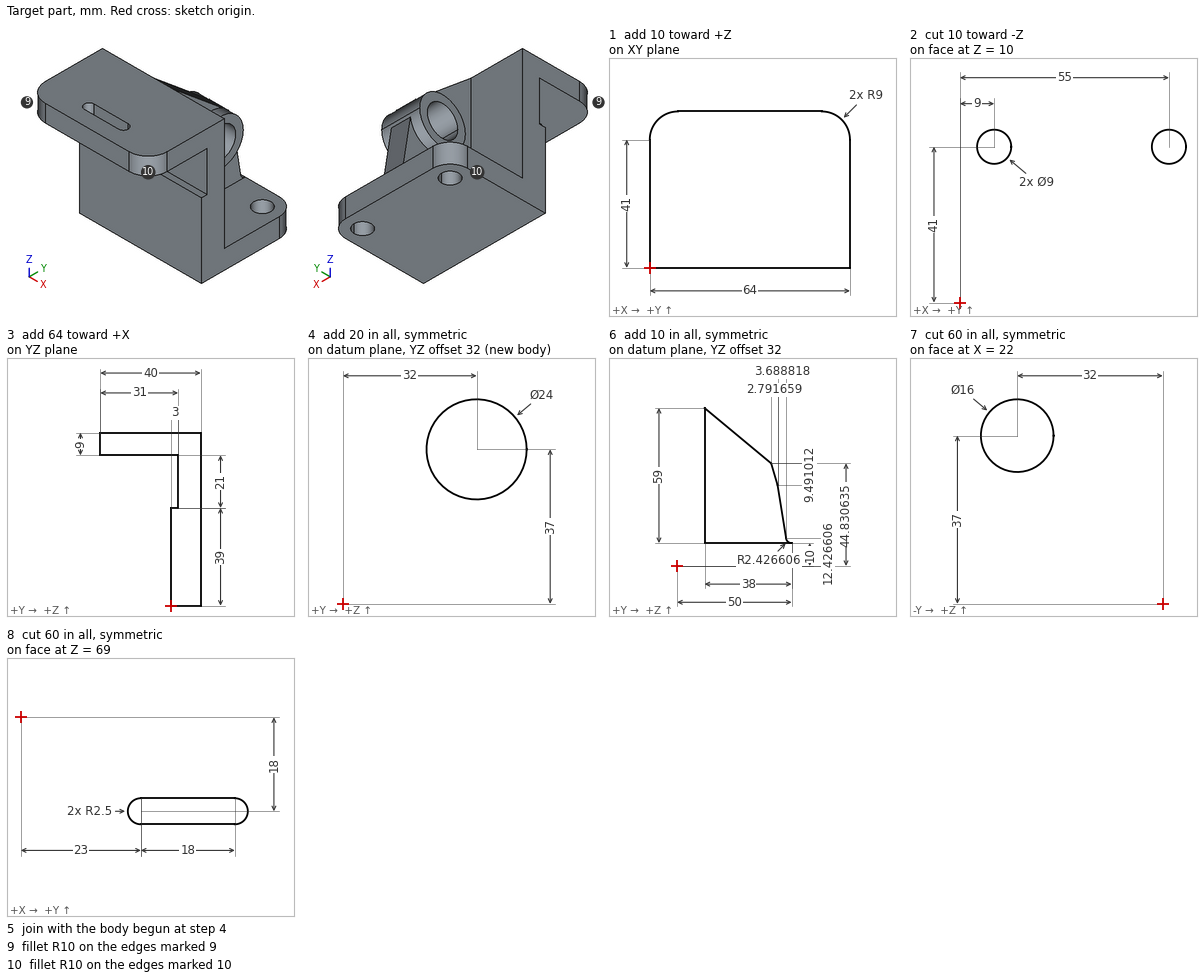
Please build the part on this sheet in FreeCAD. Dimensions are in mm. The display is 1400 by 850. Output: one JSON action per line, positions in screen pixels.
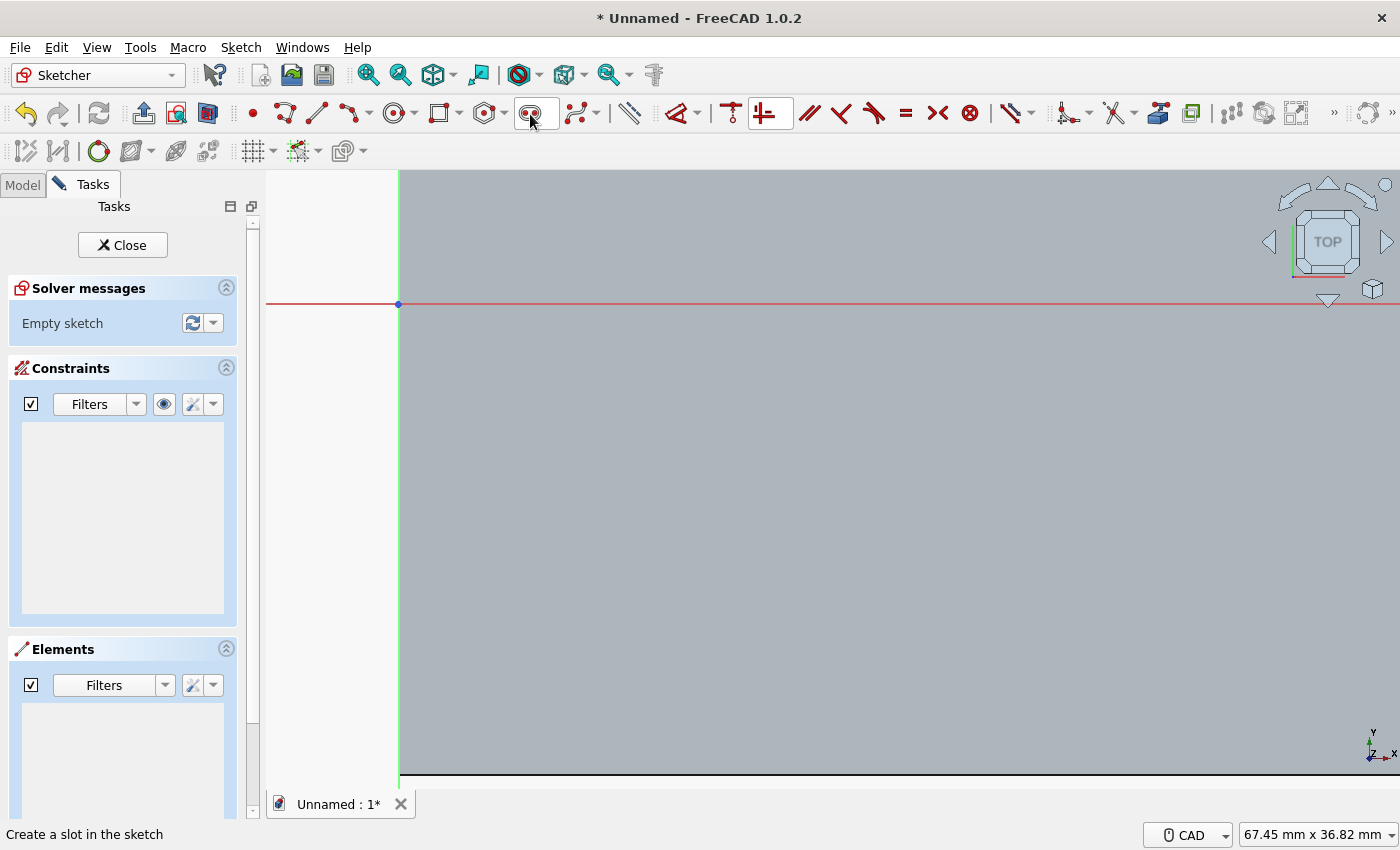
{"action": "left_click", "coordinate": [785, 607]}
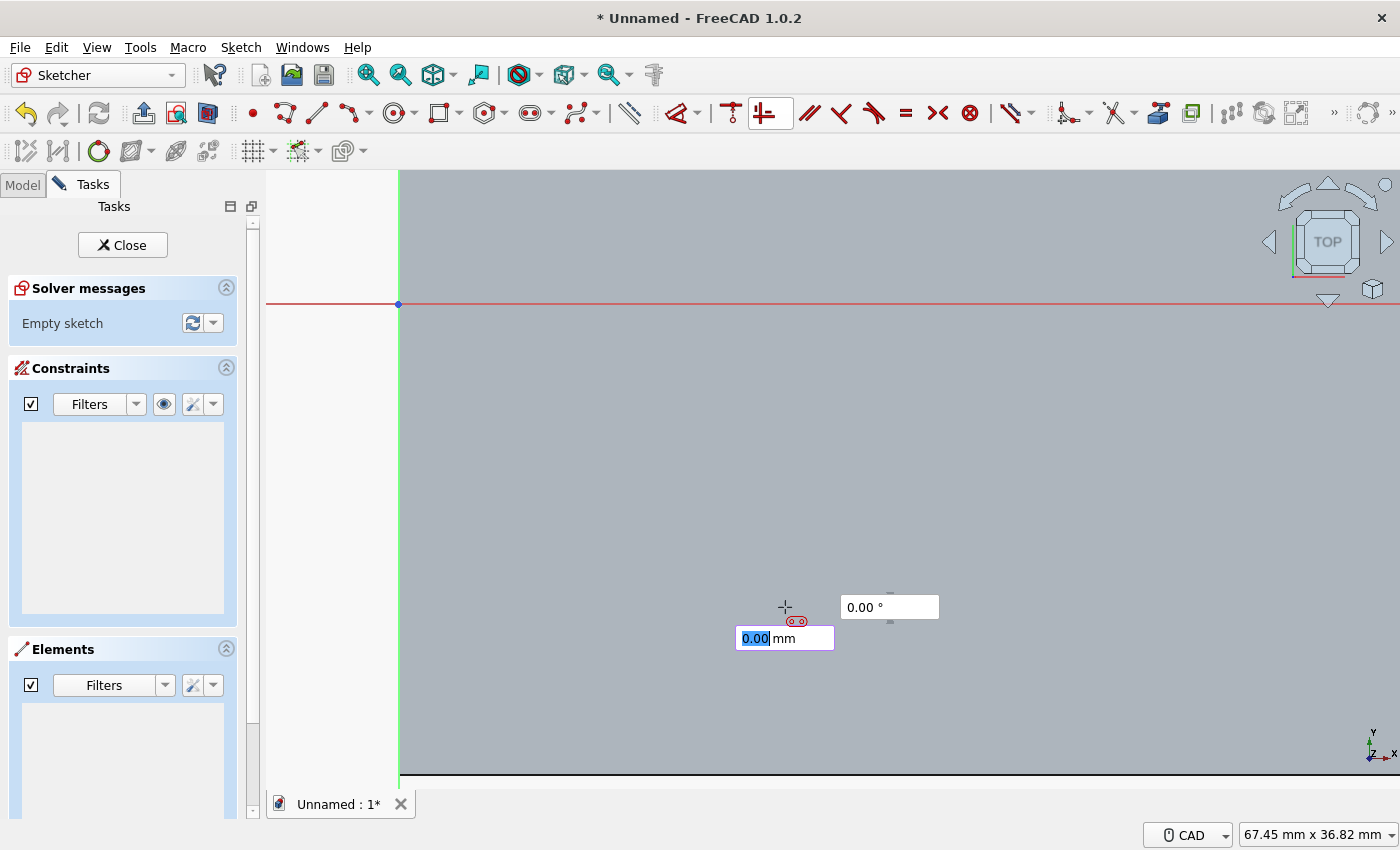
{"action": "left_click", "coordinate": [1088, 607]}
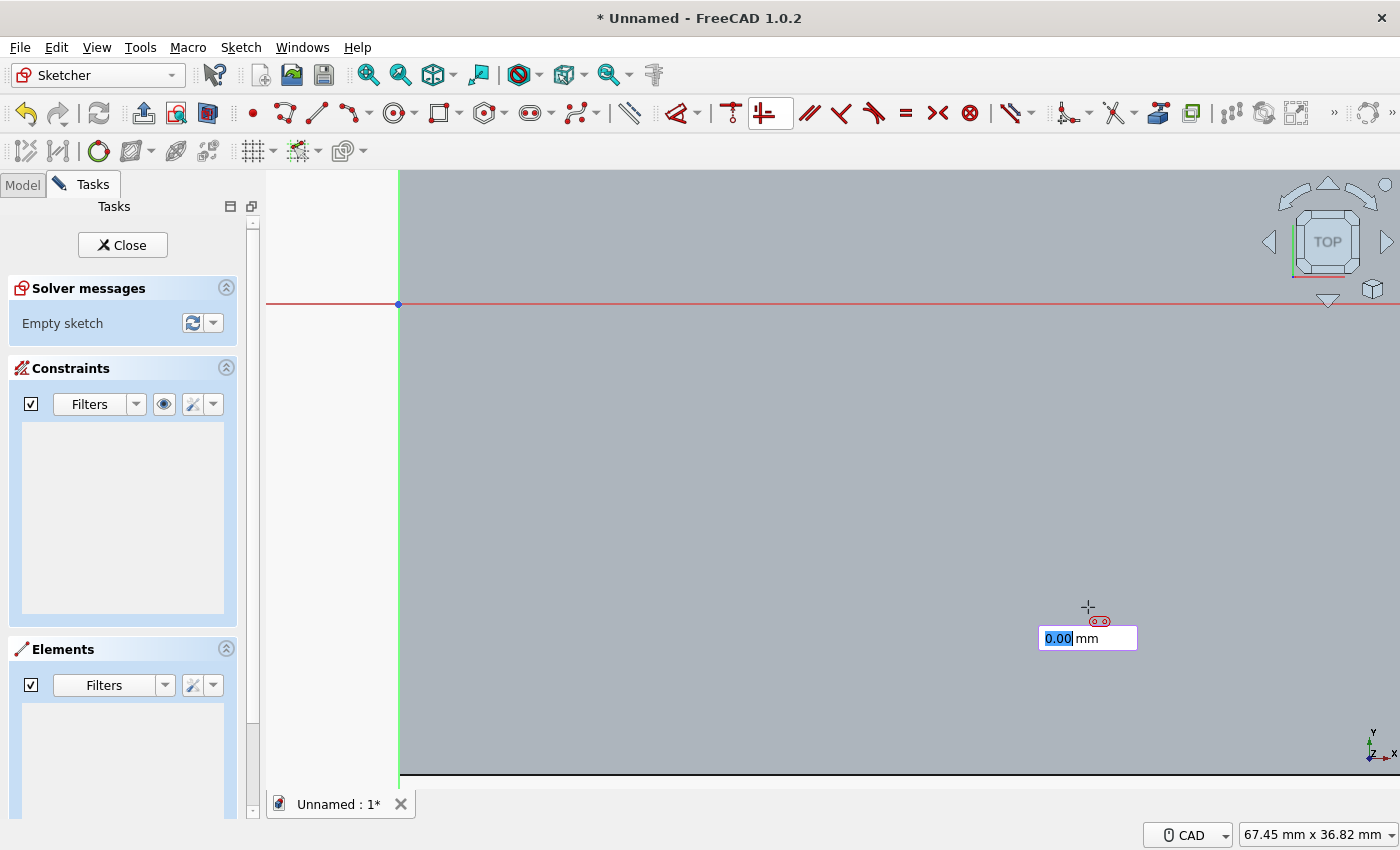
{"action": "left_click", "coordinate": [937, 565]}
{"action": "key", "text": "Escape"}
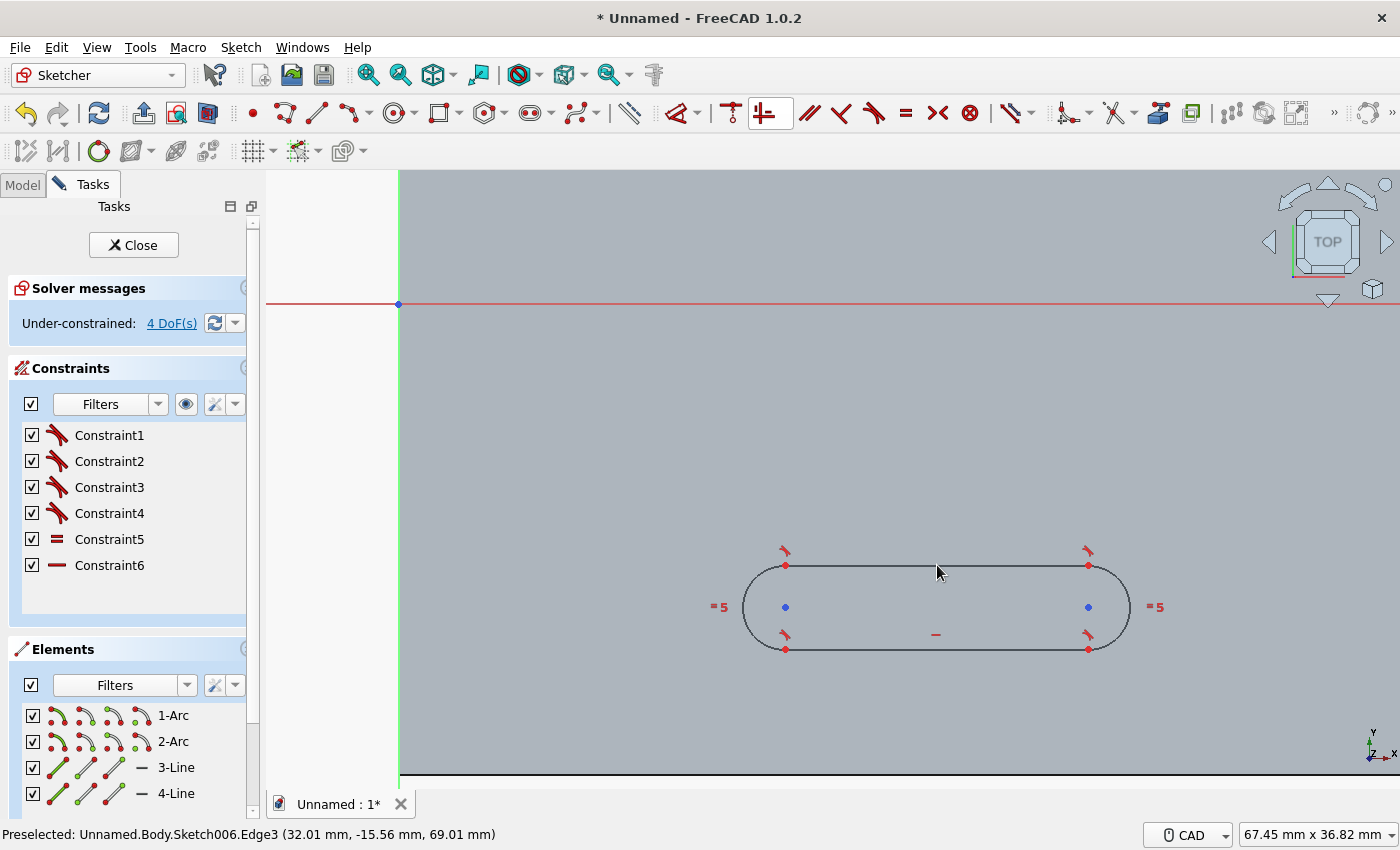
{"action": "left_click", "coordinate": [676, 114]}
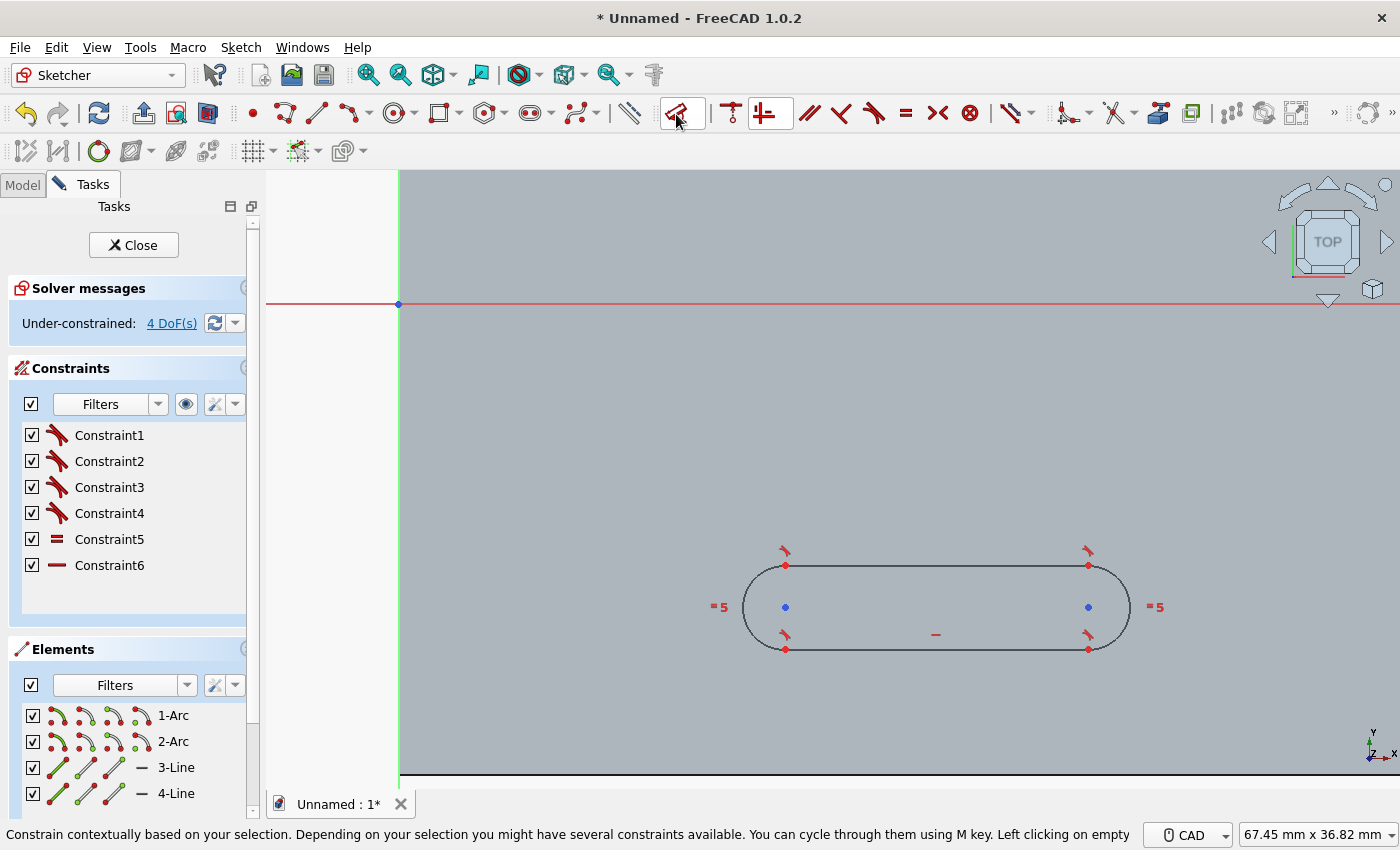
{"action": "left_click", "coordinate": [751, 583]}
{"action": "left_click", "coordinate": [725, 564]}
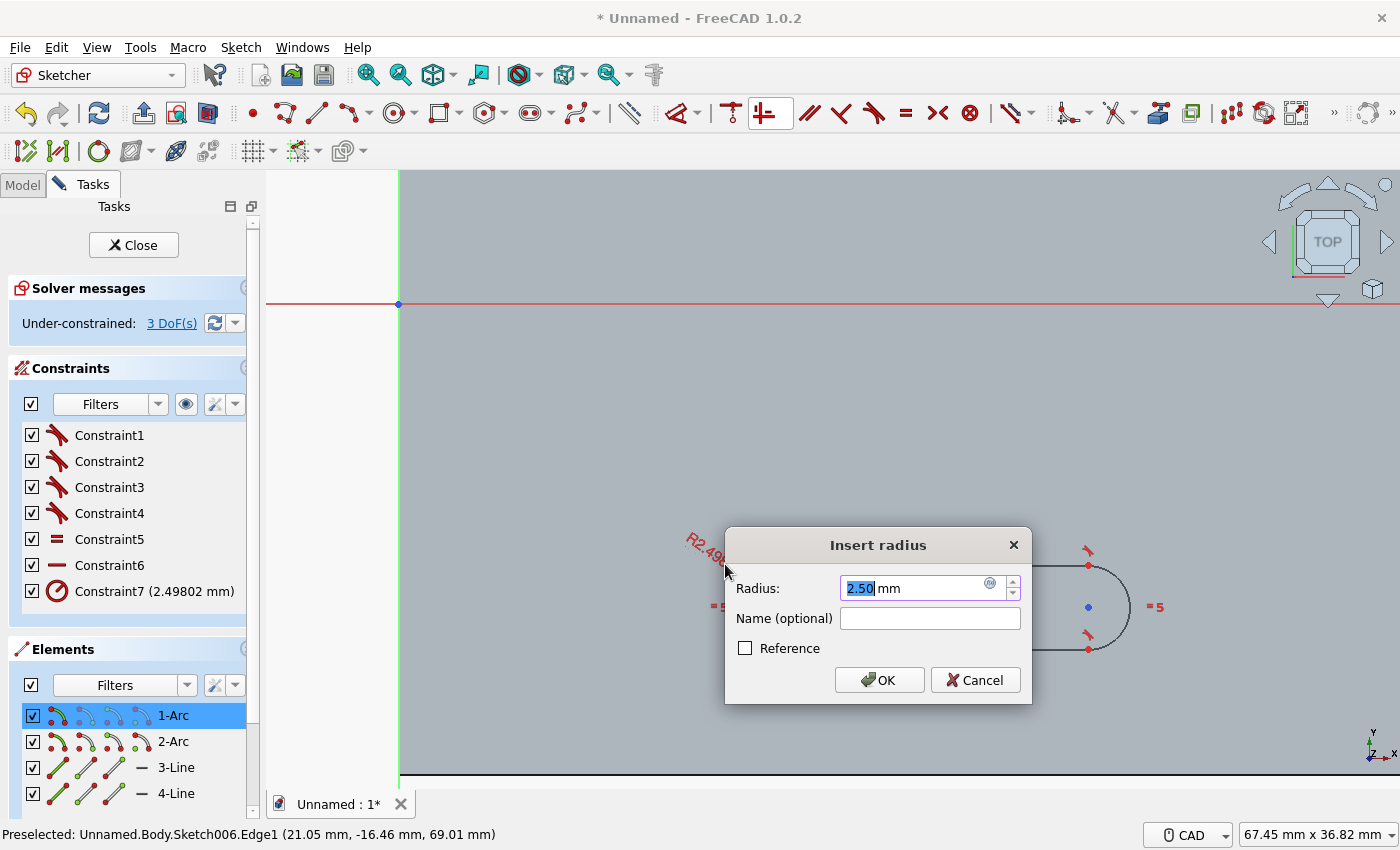
{"action": "type", "text": "2.5"}
{"action": "key", "text": "Return"}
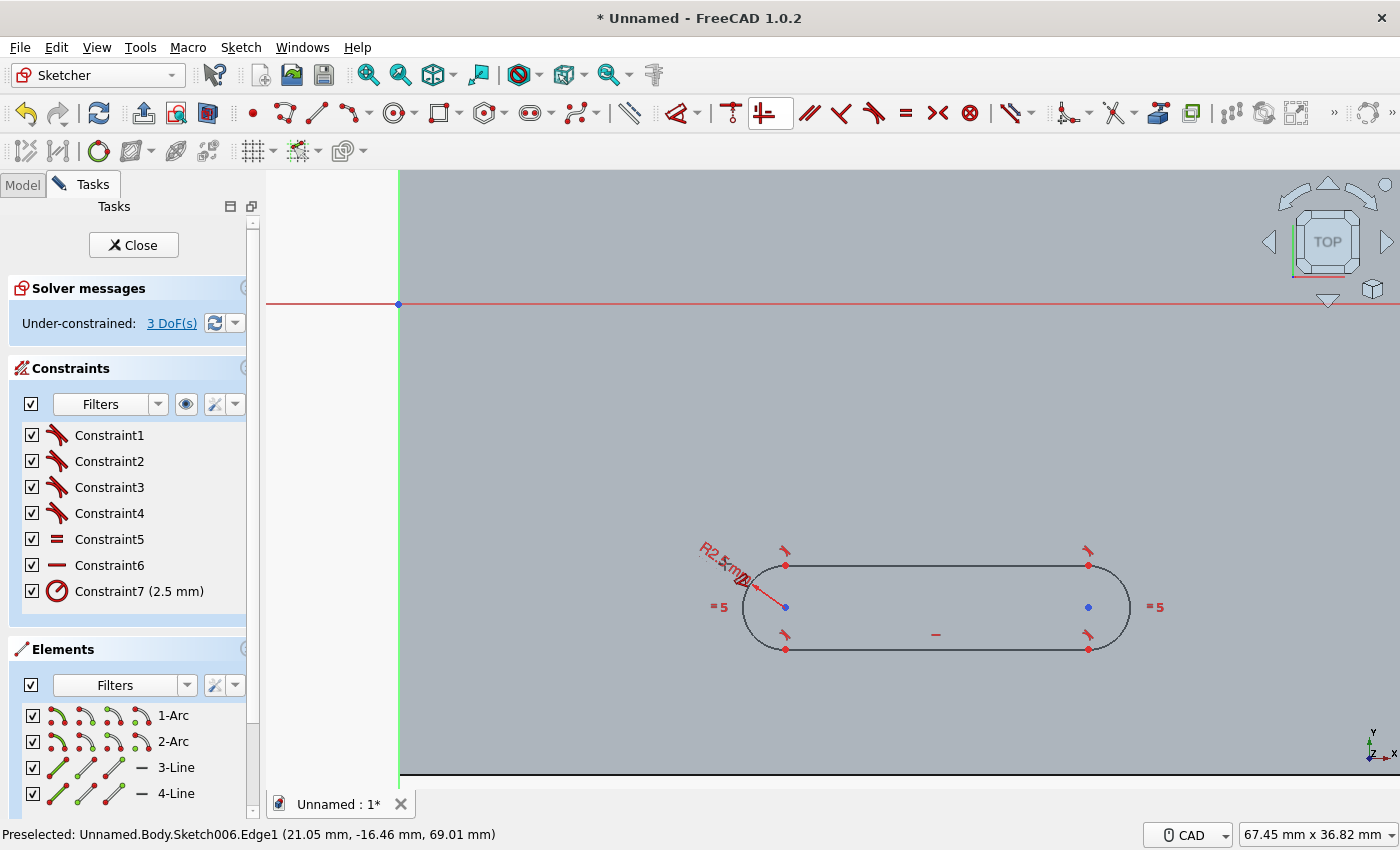
{"action": "left_click", "coordinate": [876, 566]}
{"action": "left_click", "coordinate": [937, 600]}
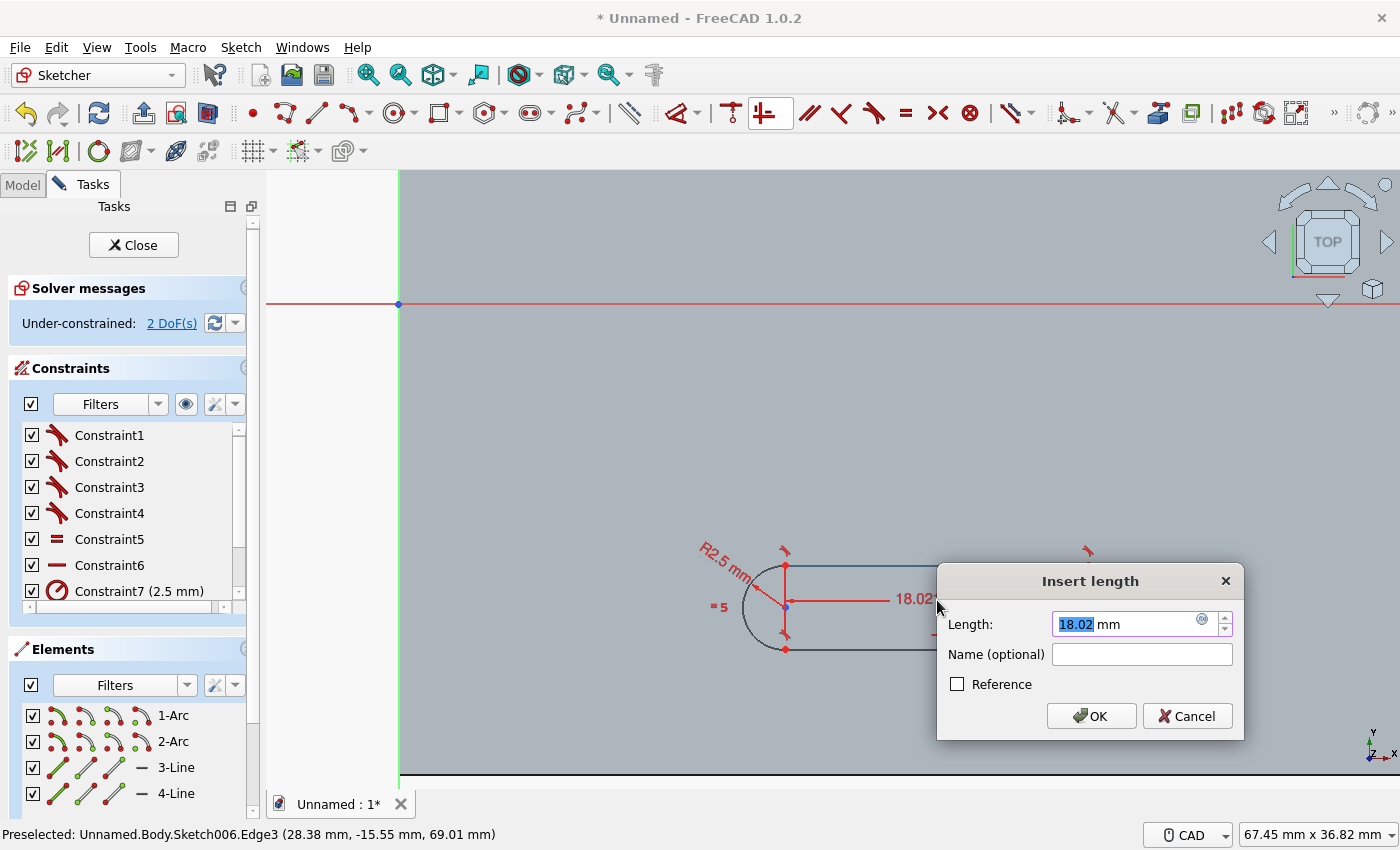
{"action": "type", "text": "18"}
{"action": "key", "text": "Return"}